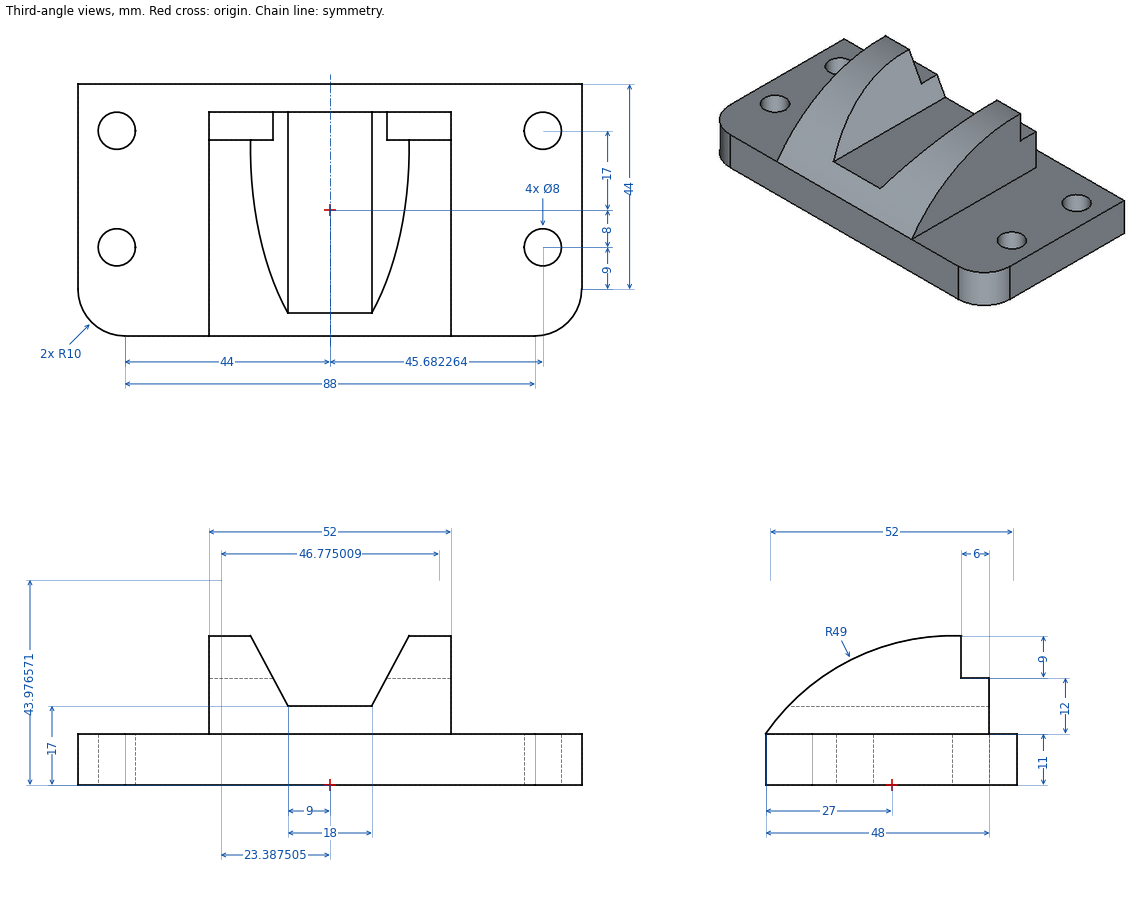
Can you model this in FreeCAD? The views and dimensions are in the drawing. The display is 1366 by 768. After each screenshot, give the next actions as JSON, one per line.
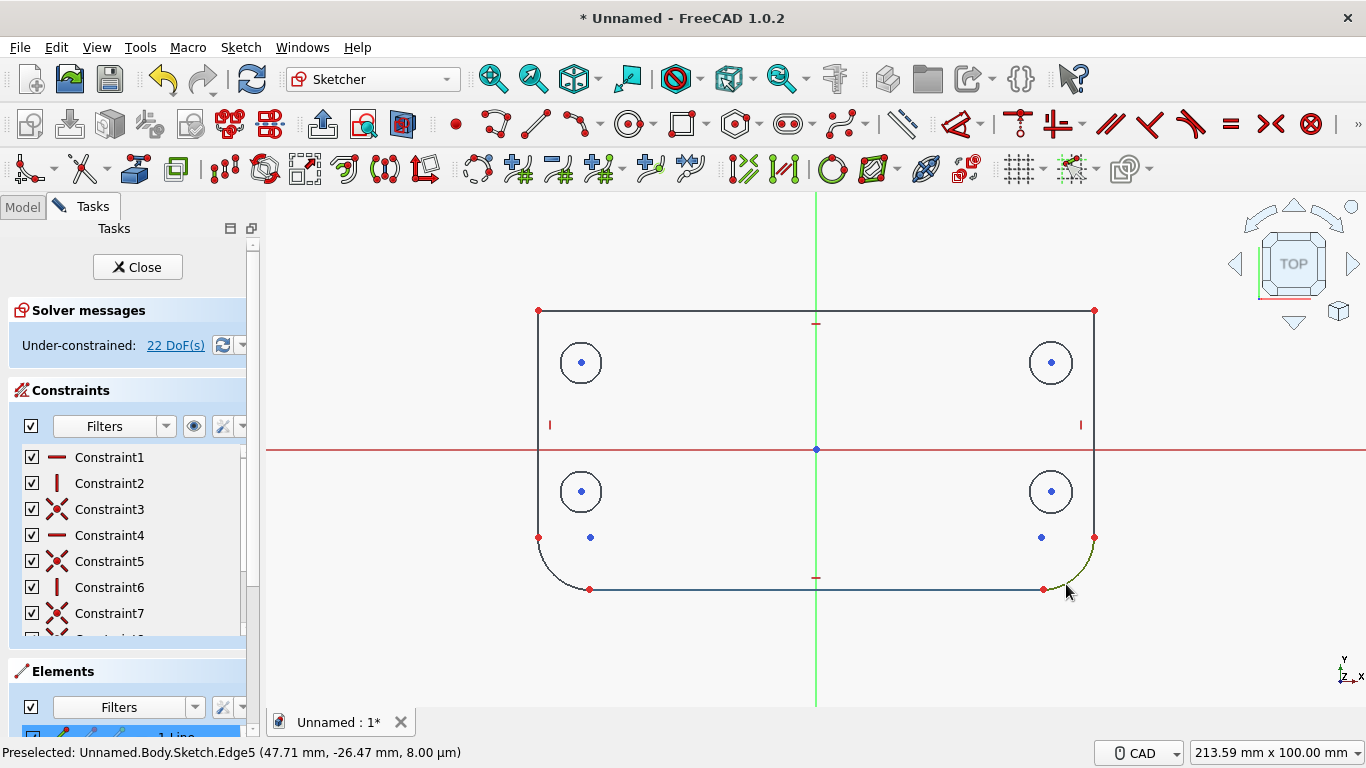
{"action": "key", "text": "t"}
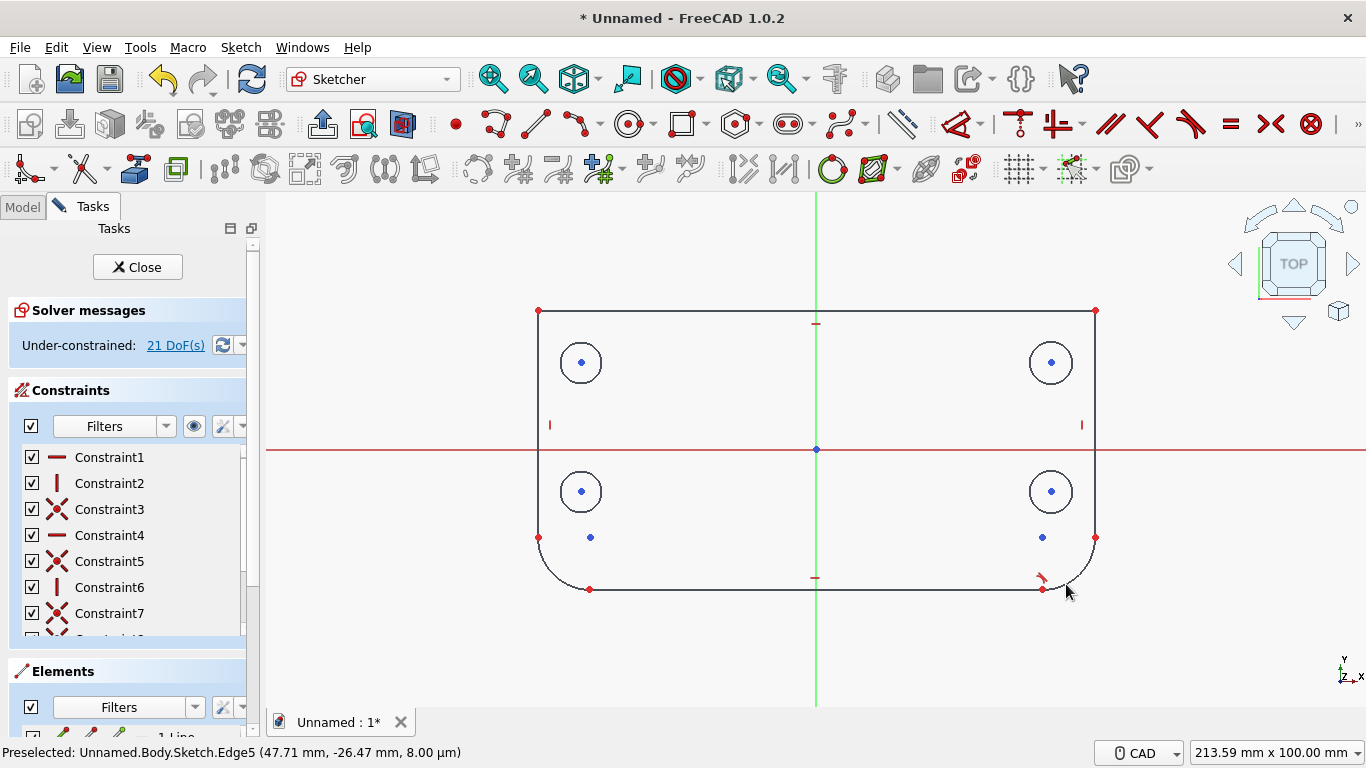
{"action": "left_click", "coordinate": [725, 590]}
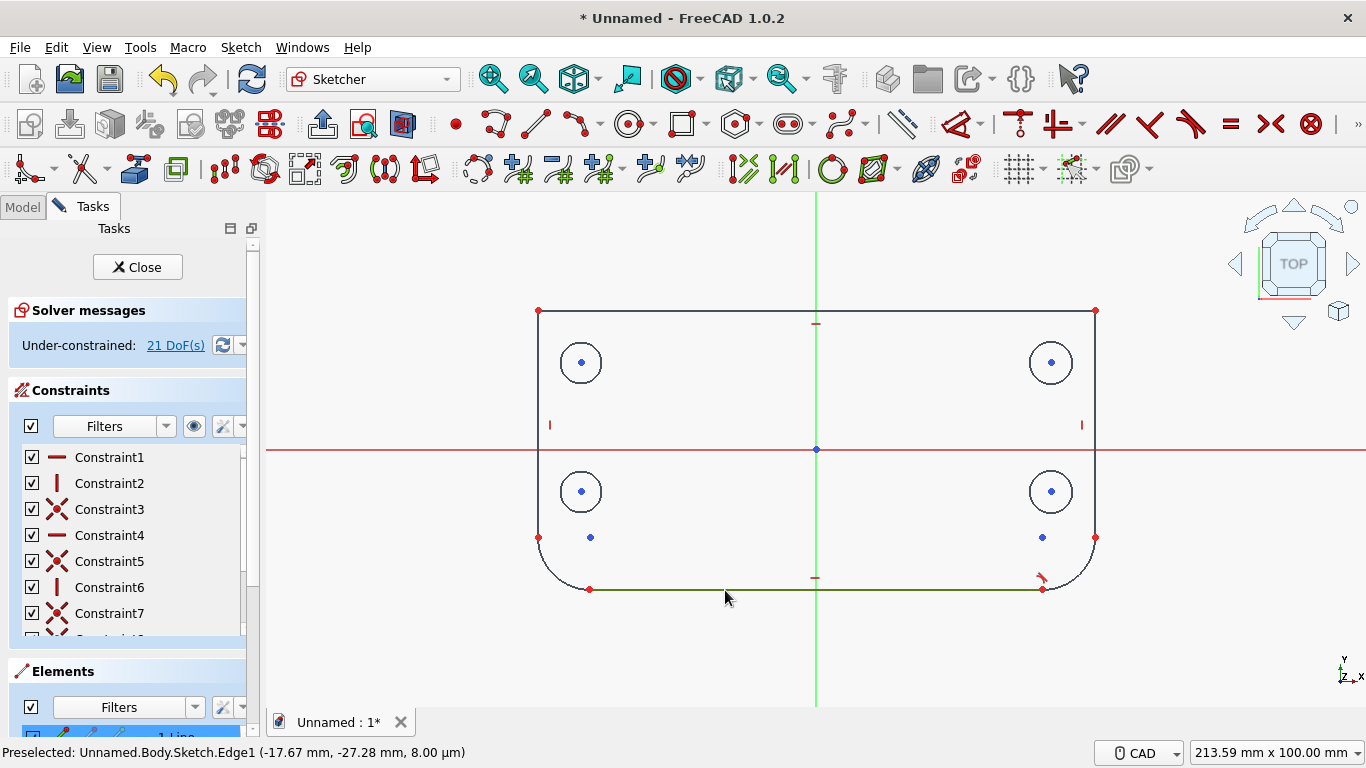
{"action": "left_click", "coordinate": [544, 561]}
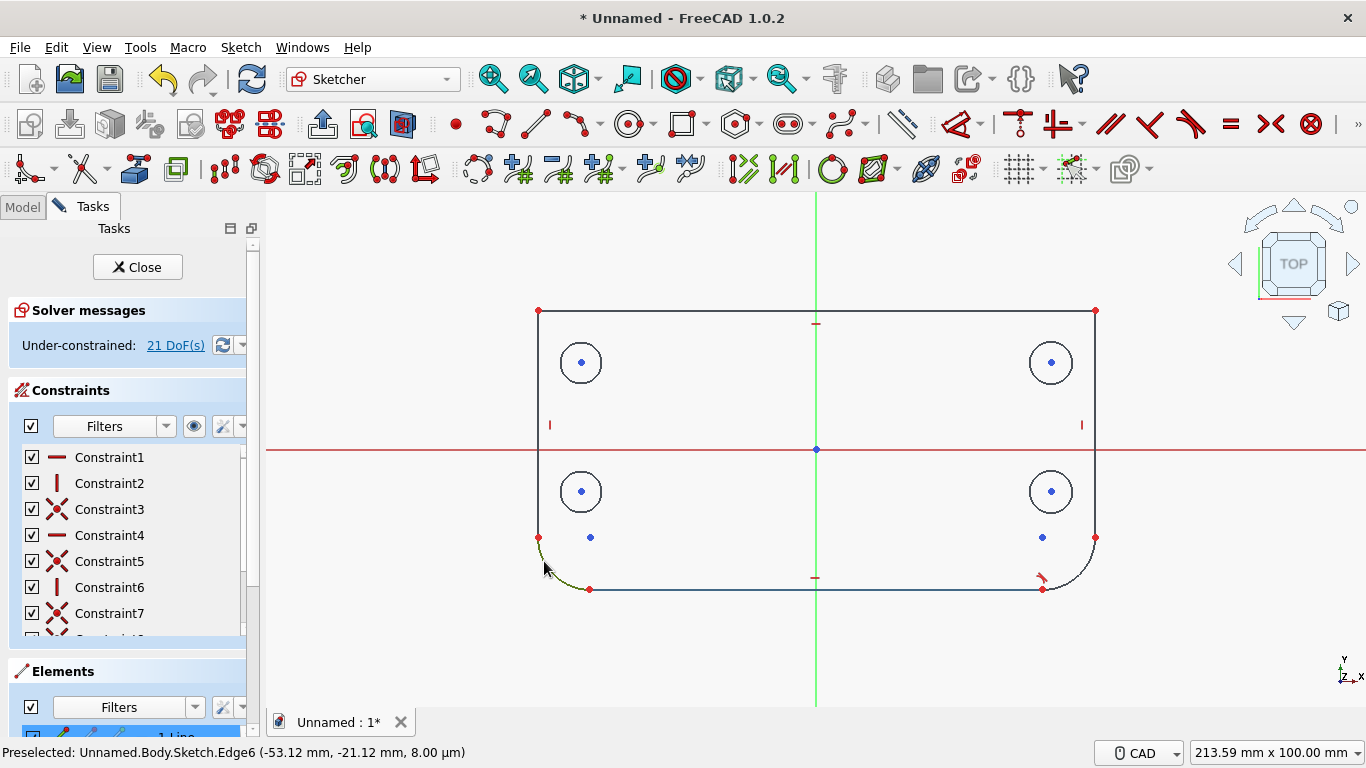
{"action": "key", "text": "t"}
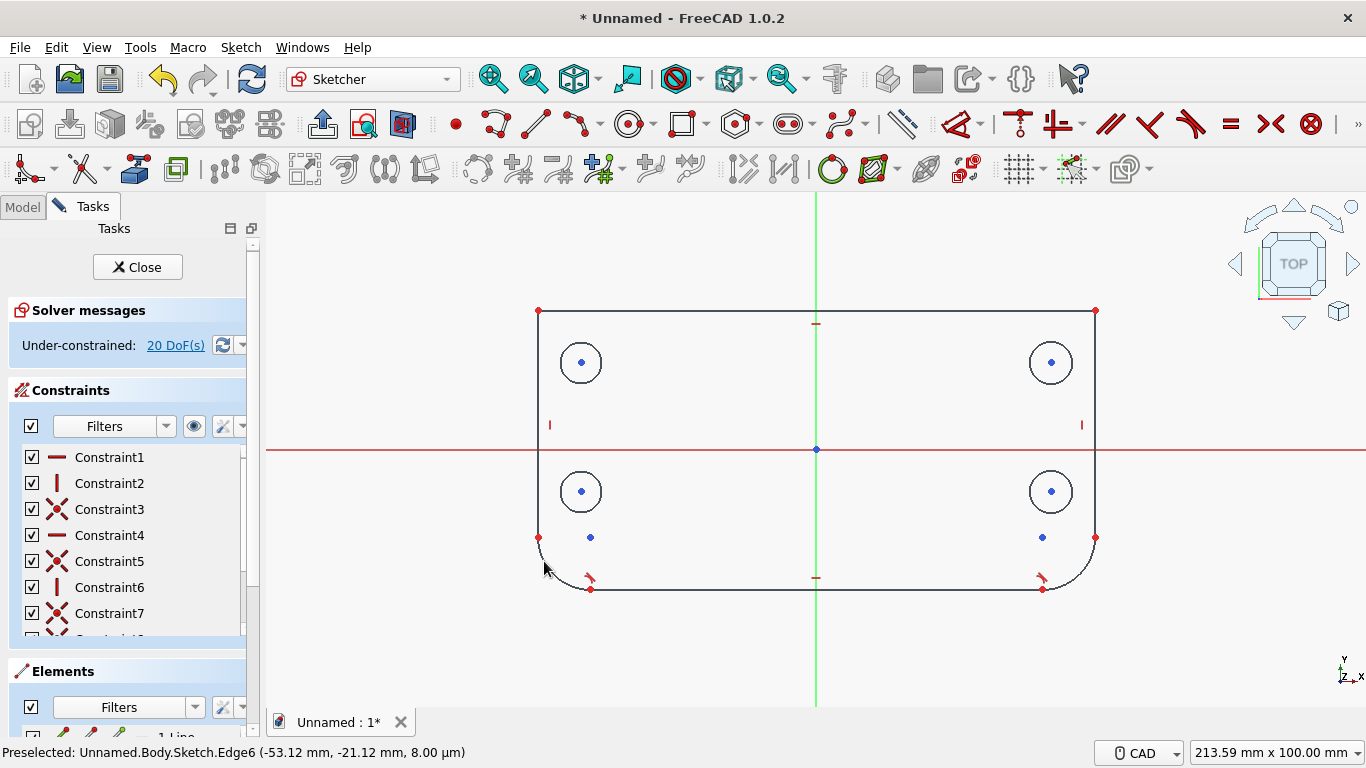
{"action": "left_click", "coordinate": [1095, 470]}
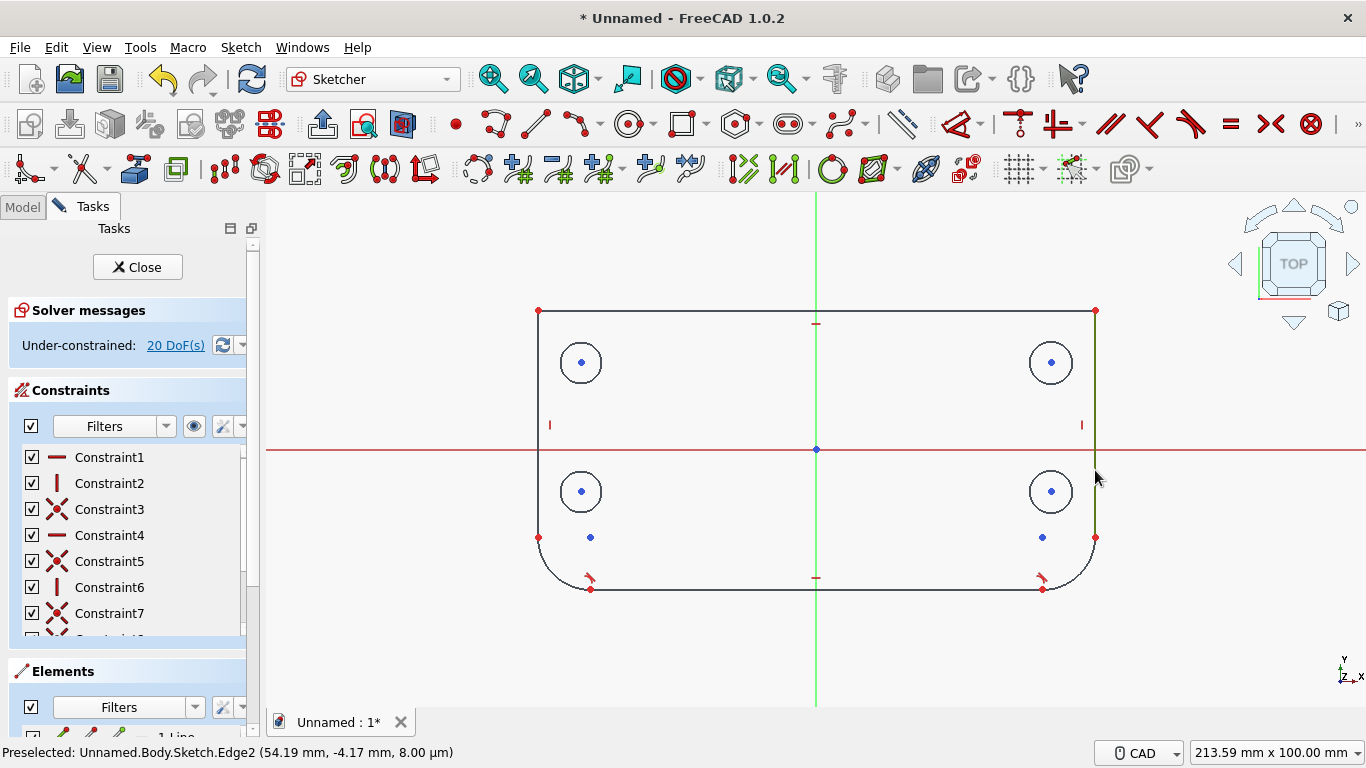
{"action": "left_click", "coordinate": [1066, 584]}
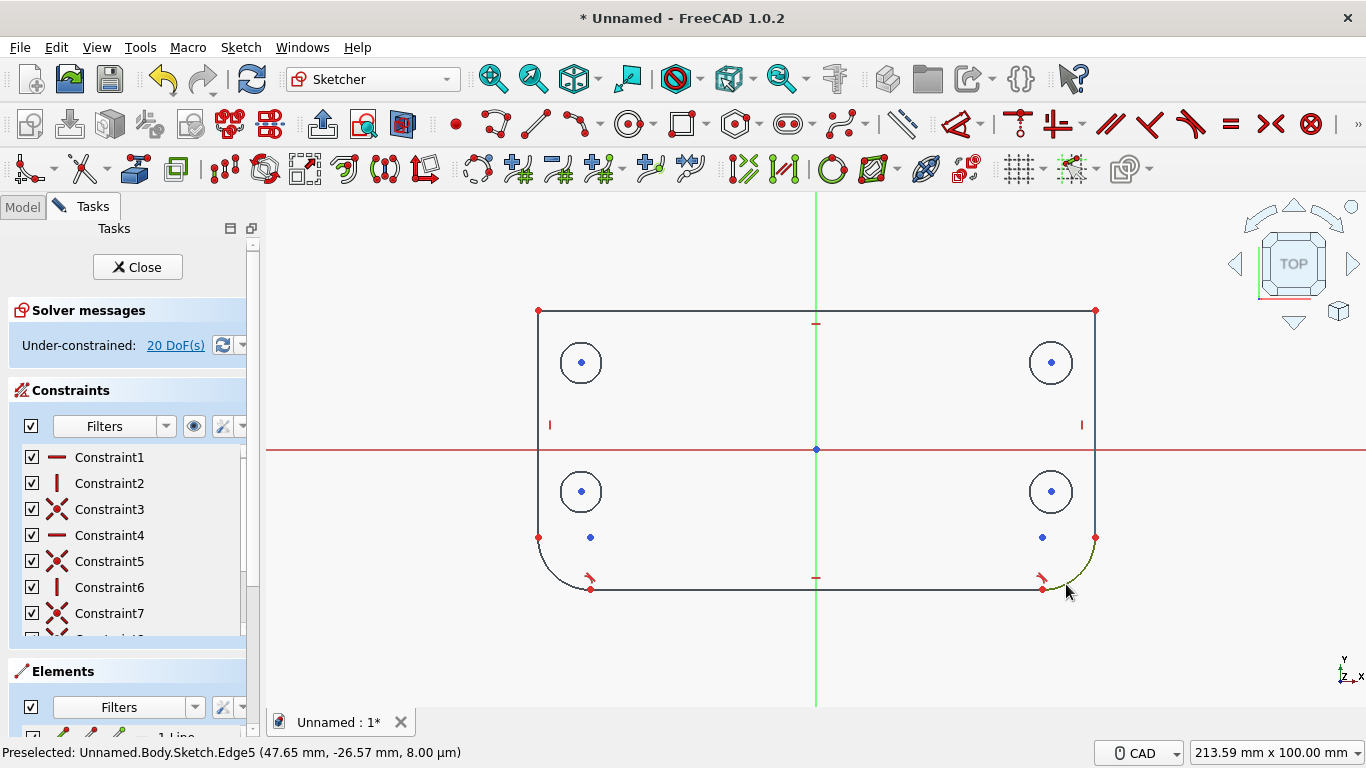
{"action": "key", "text": "t"}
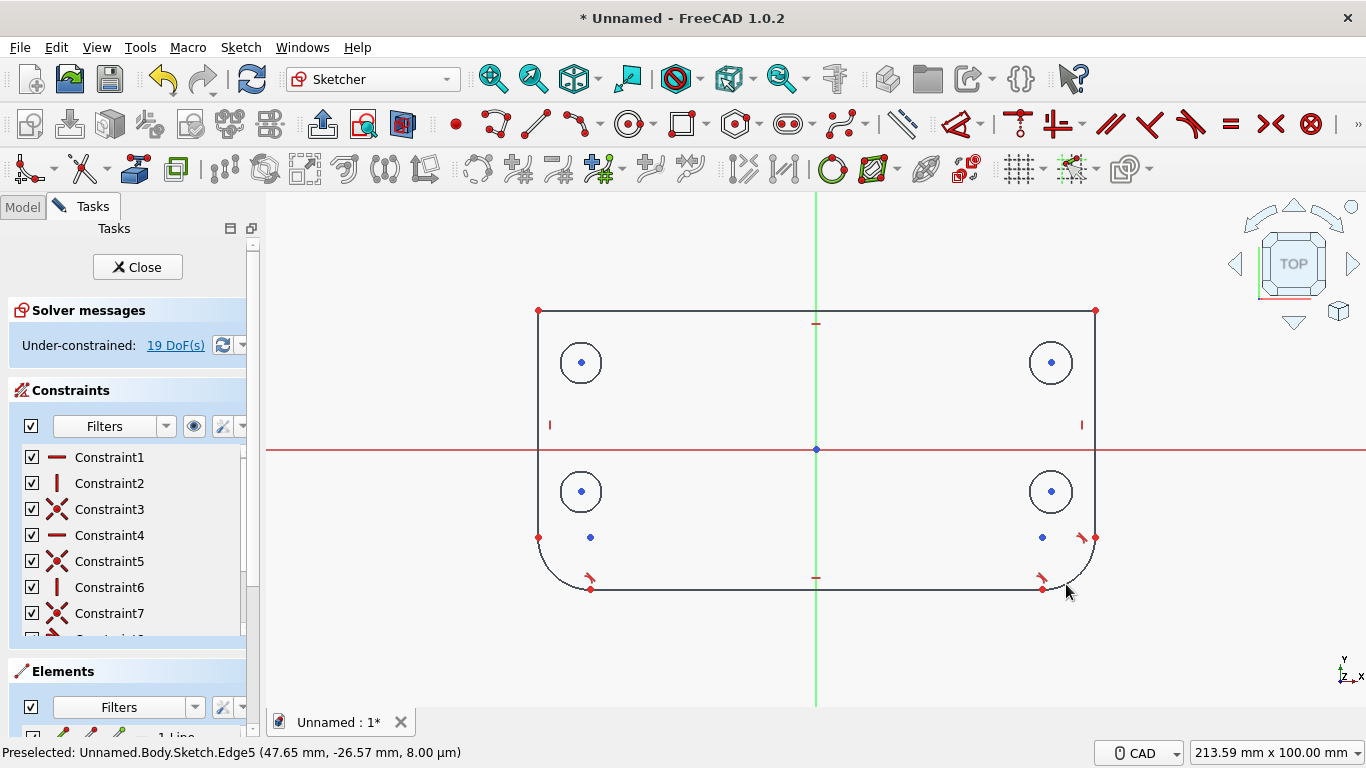
{"action": "left_click", "coordinate": [538, 379]}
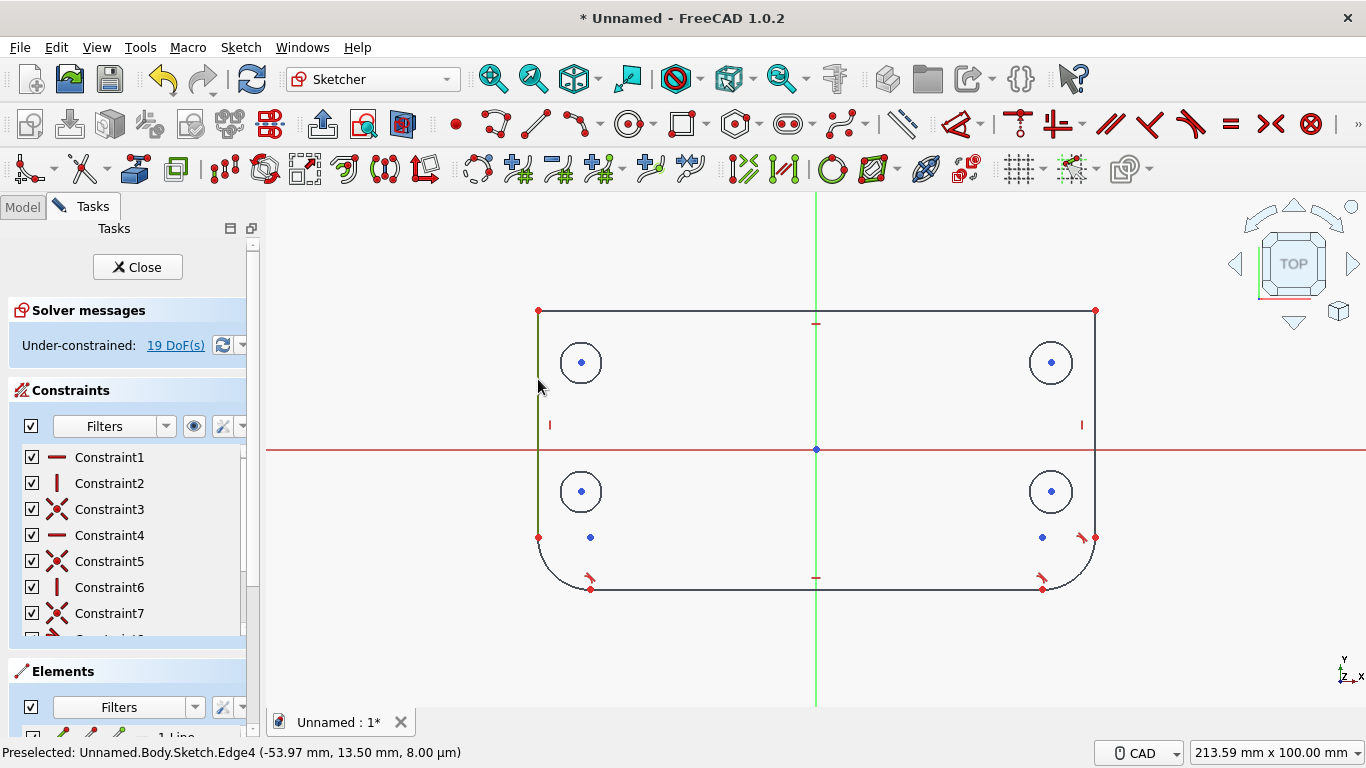
{"action": "left_click", "coordinate": [544, 562]}